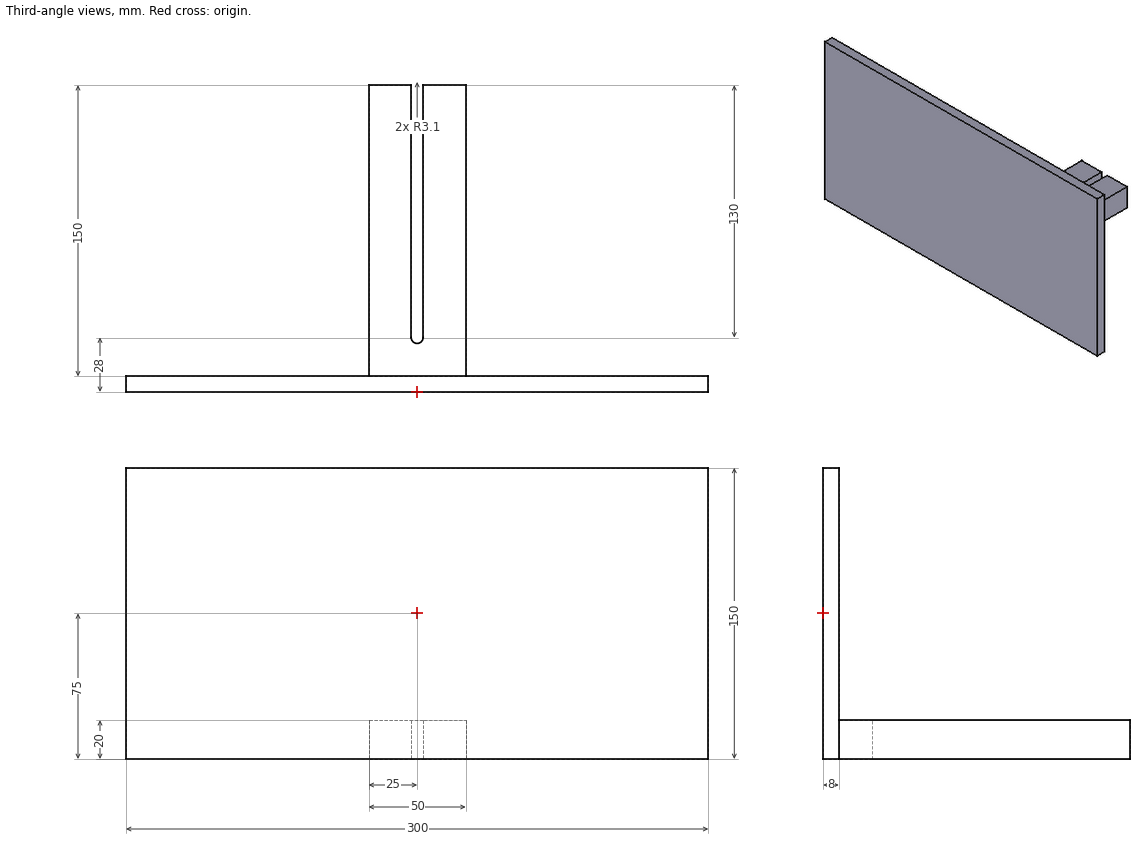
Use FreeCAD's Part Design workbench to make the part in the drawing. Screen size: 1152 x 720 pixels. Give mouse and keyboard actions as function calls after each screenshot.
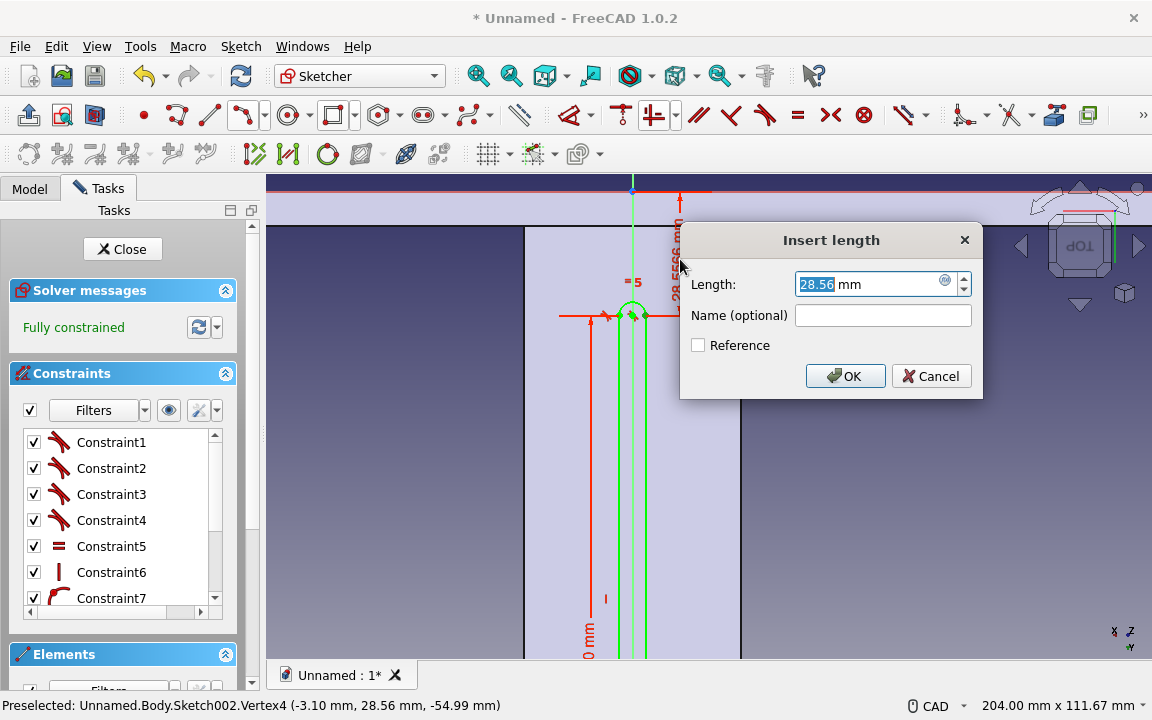
text(28)
key(Return)
key(Escape)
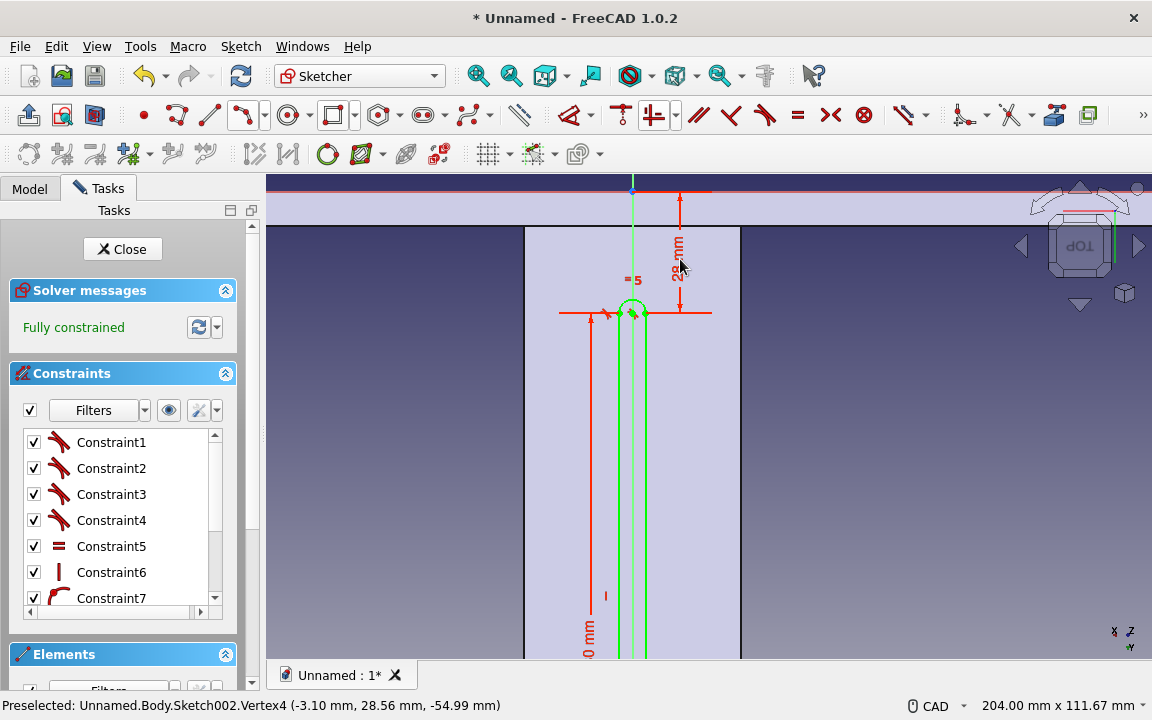
click(123, 249)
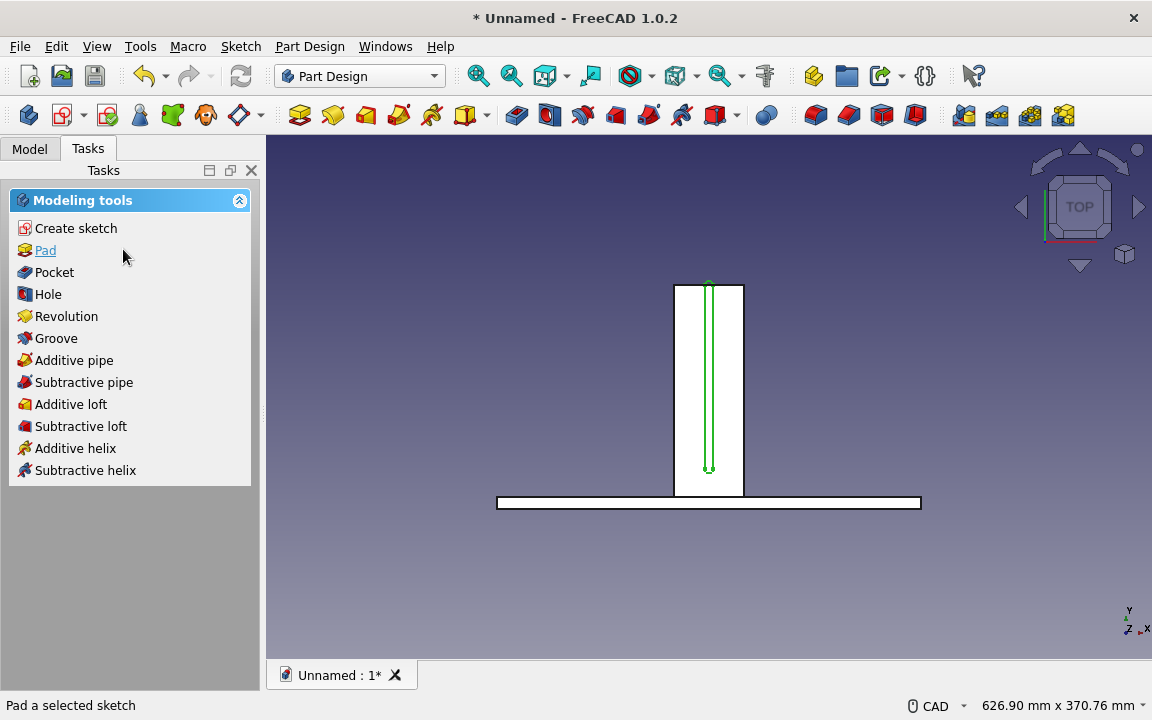
click(517, 116)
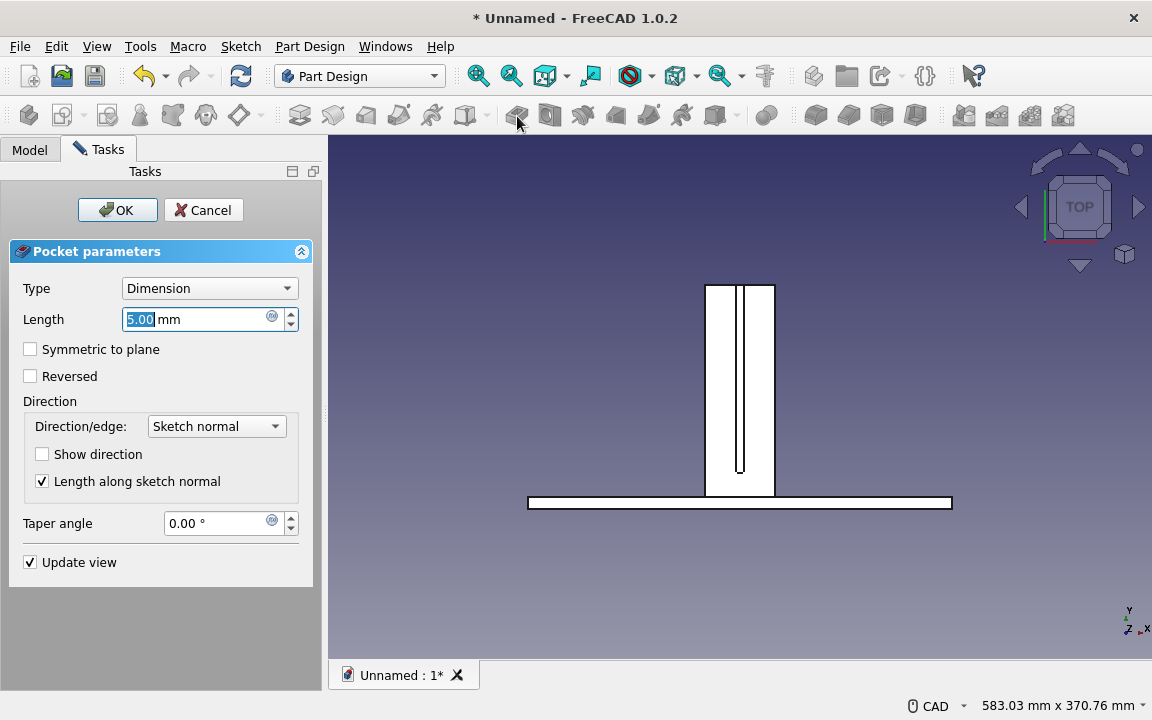
click(210, 288)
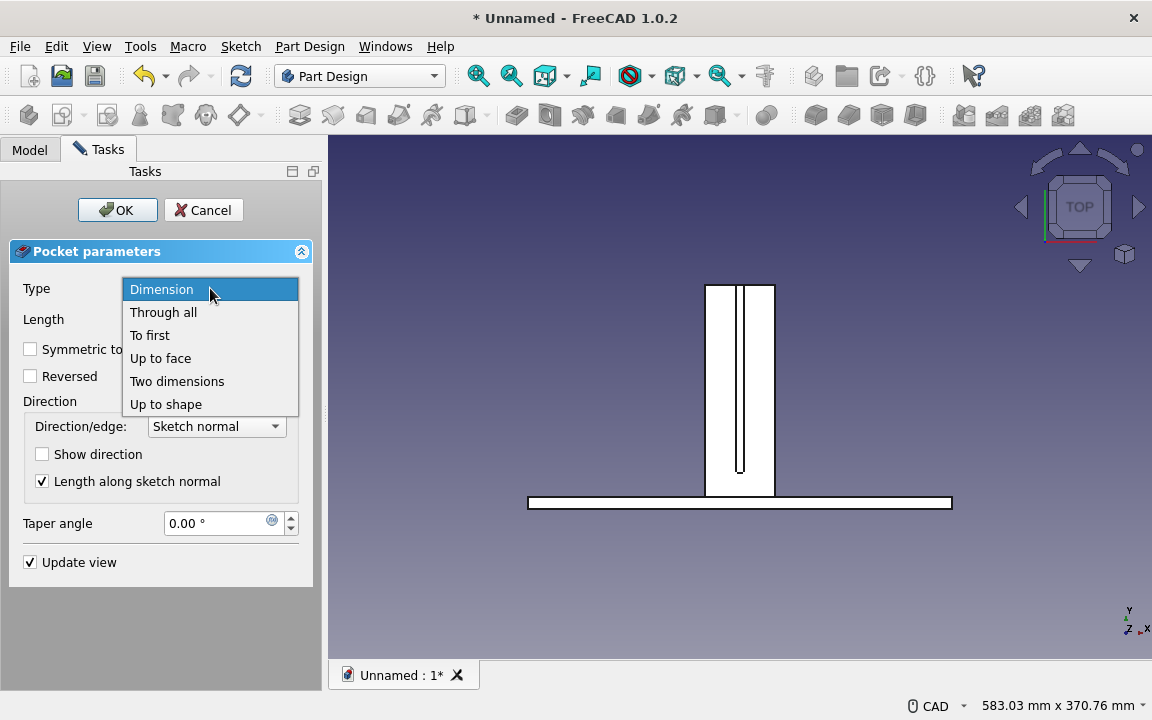
click(208, 312)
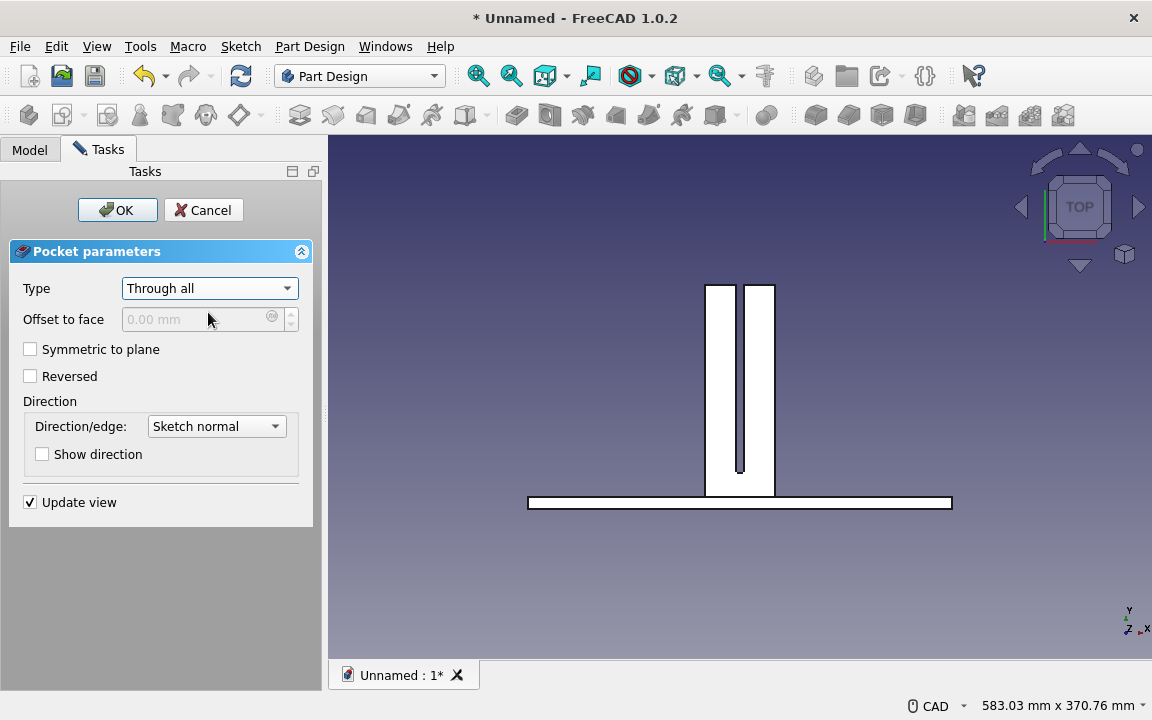
click(118, 210)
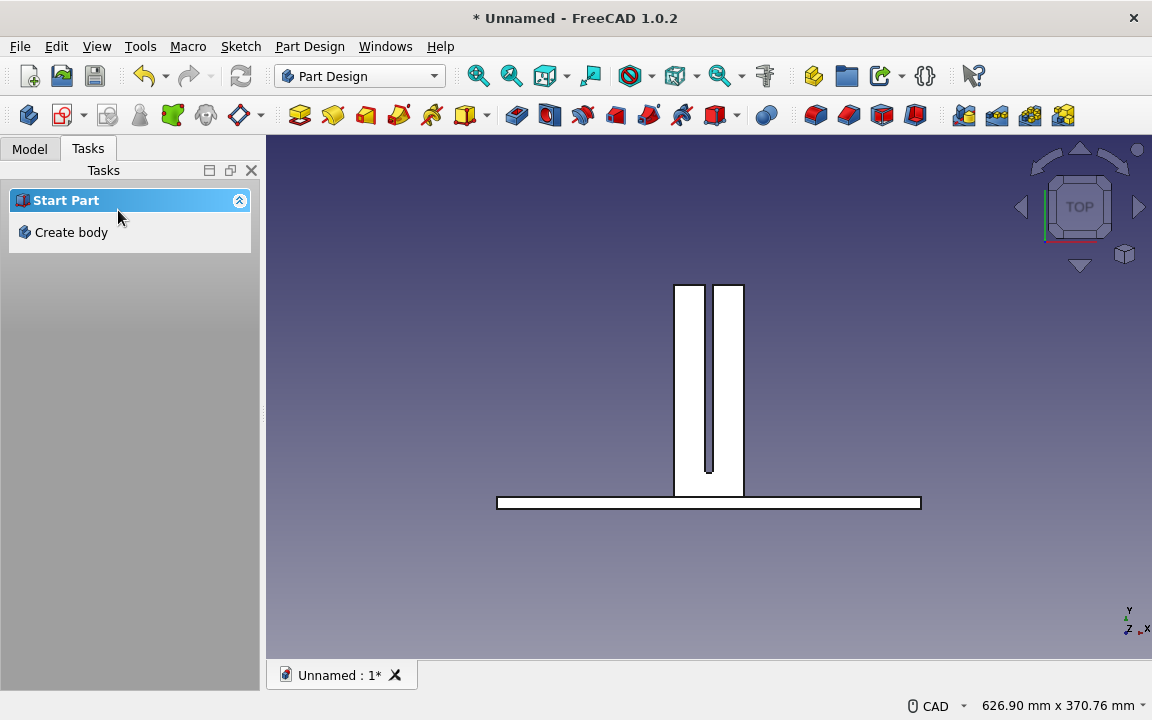
key(0)